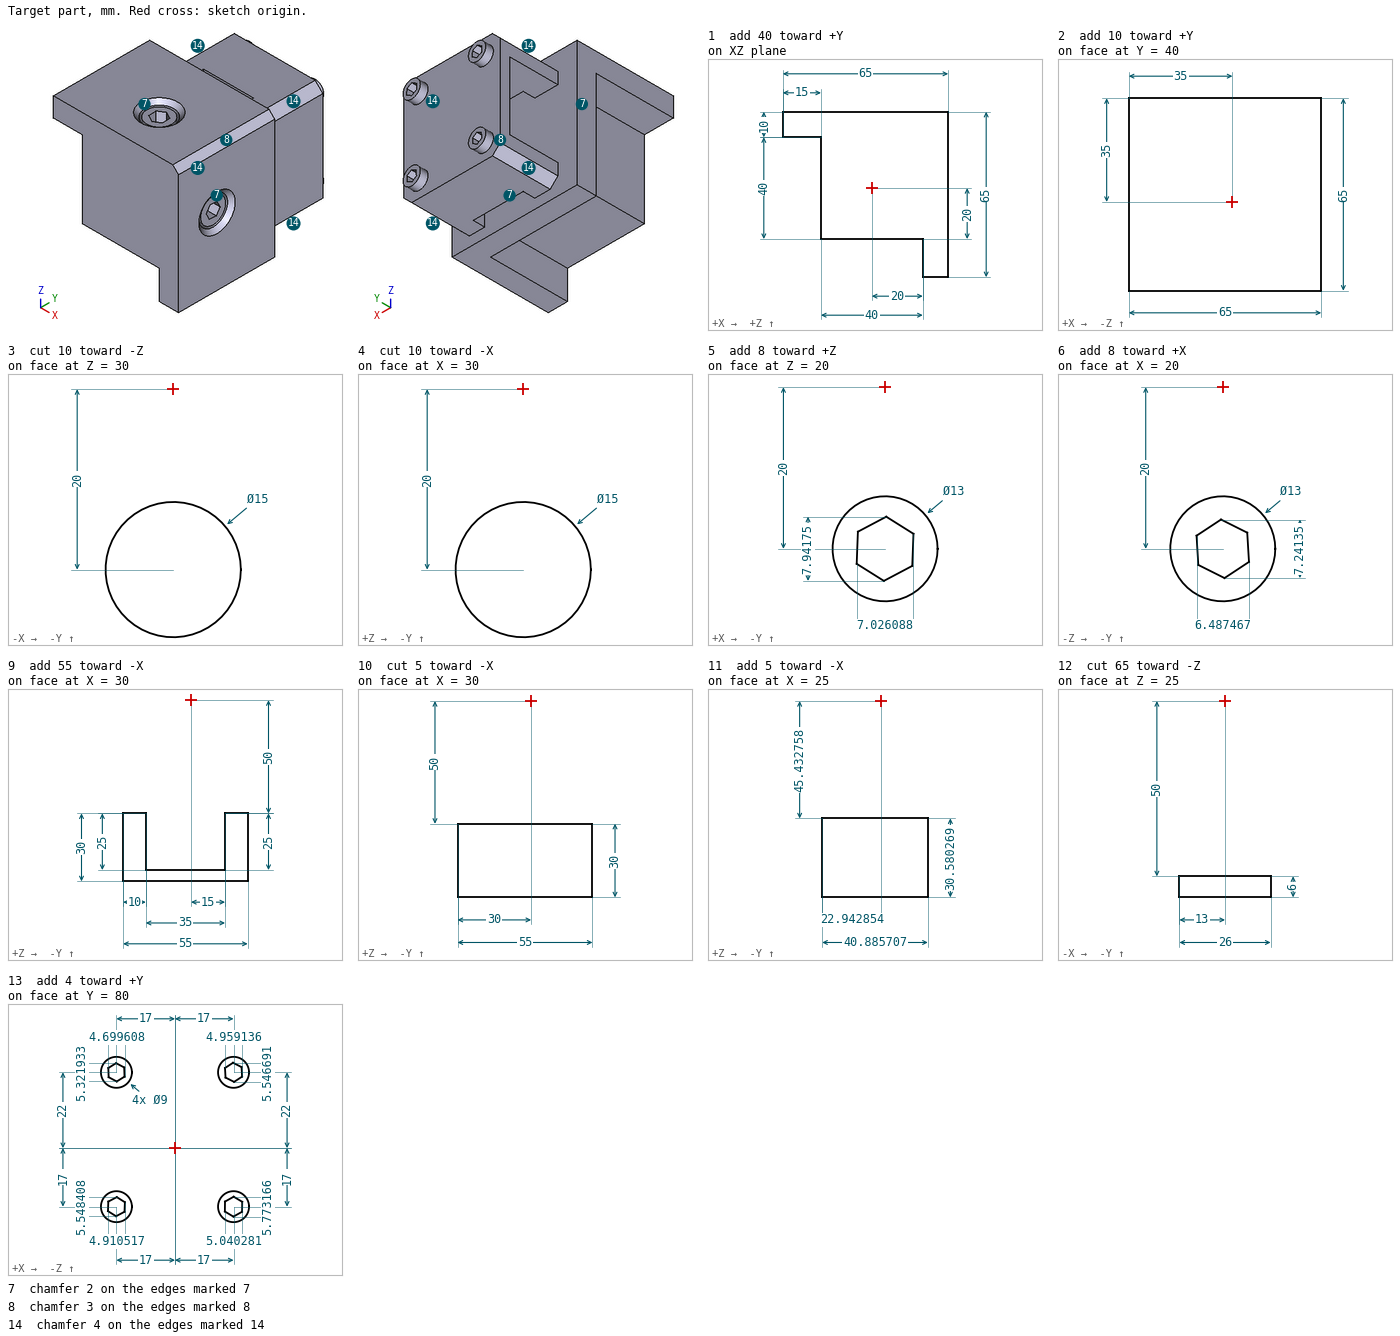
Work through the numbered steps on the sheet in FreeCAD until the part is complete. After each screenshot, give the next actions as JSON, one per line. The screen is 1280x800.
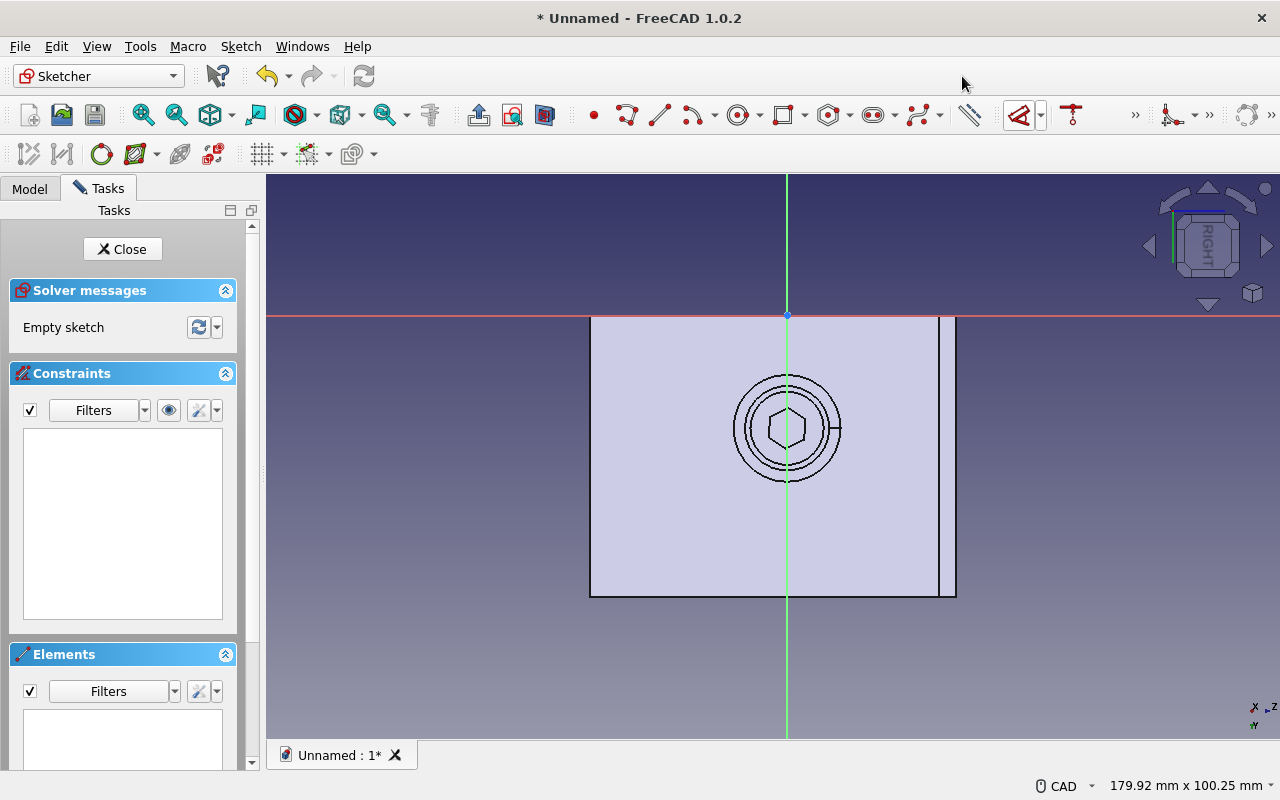
{"action": "scroll", "coordinate": [395, 202], "scroll_direction": "down", "scroll_amount": 1}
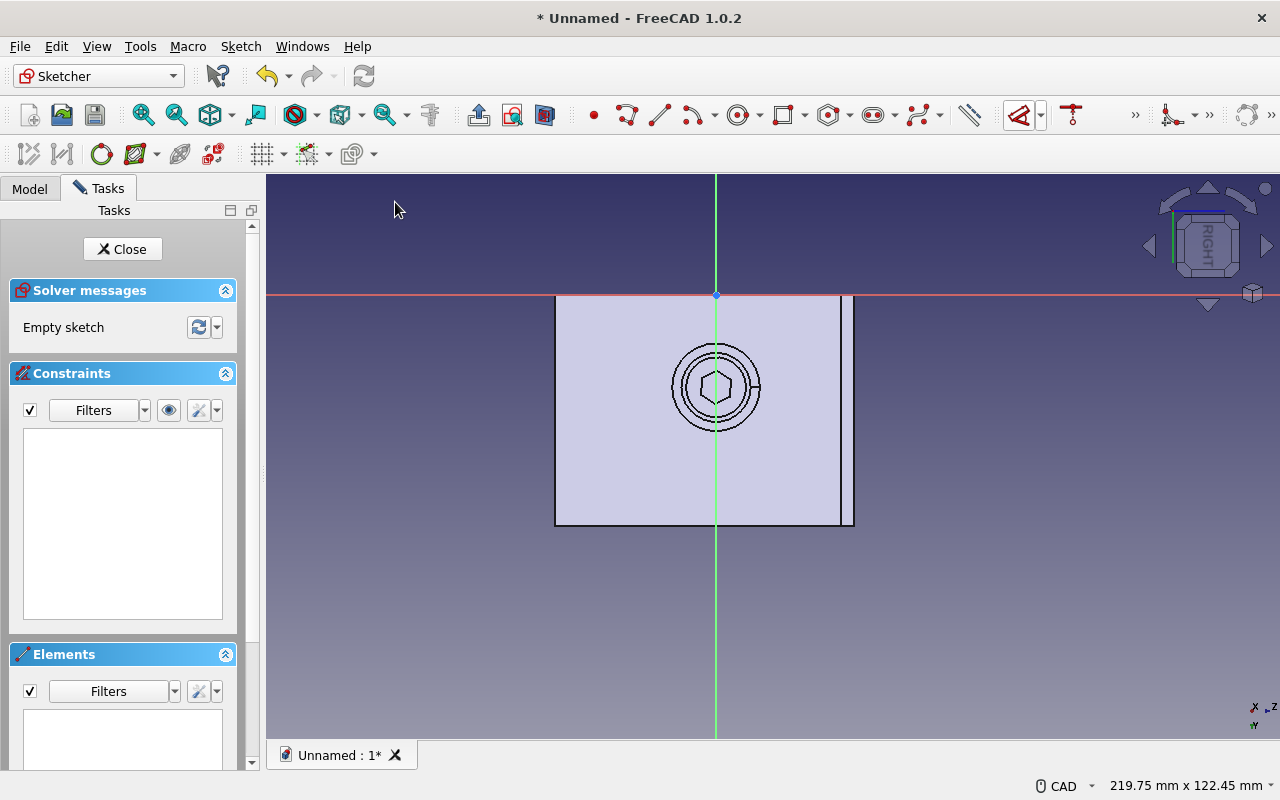
{"action": "left_click", "coordinate": [627, 116]}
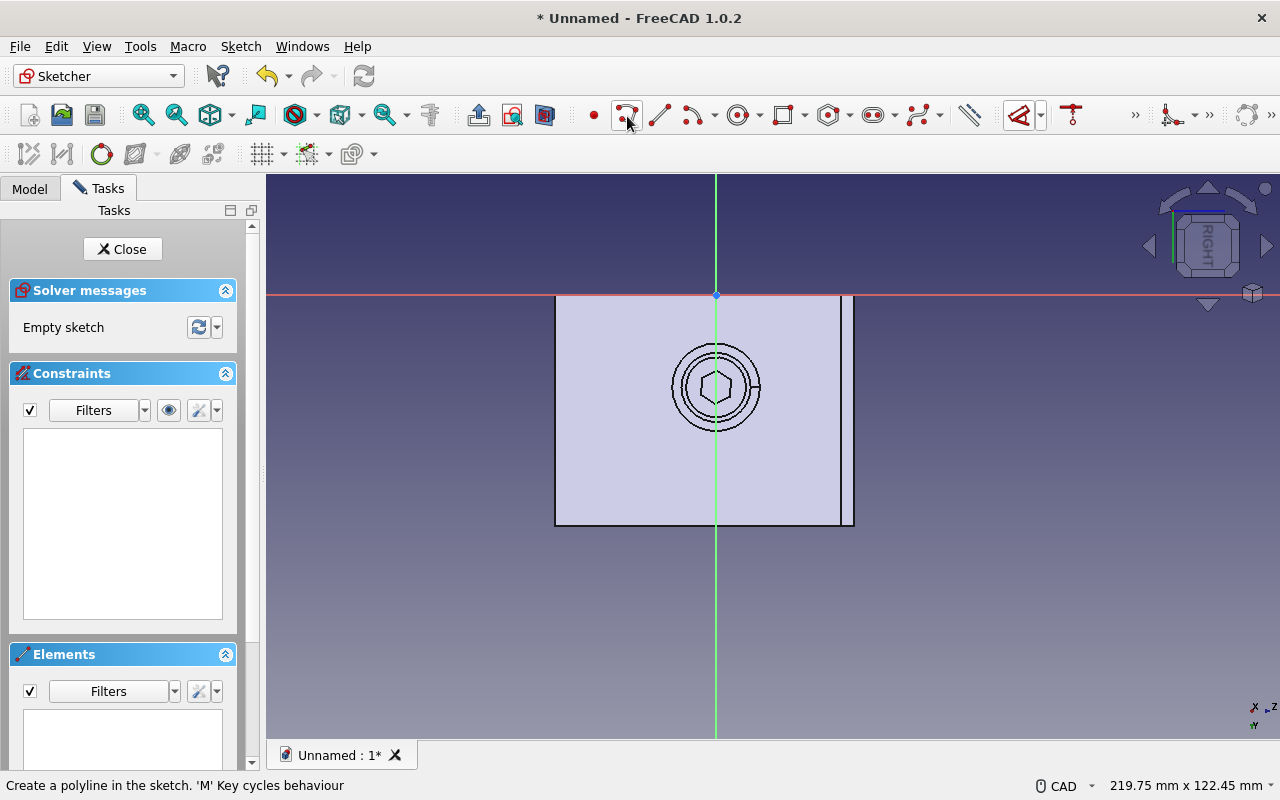
{"action": "left_click", "coordinate": [785, 526]}
{"action": "left_click", "coordinate": [785, 641]}
{"action": "left_click", "coordinate": [624, 641]}
{"action": "left_click", "coordinate": [624, 526]}
{"action": "left_click", "coordinate": [578, 526]}
{"action": "left_click", "coordinate": [578, 664]}
{"action": "left_click", "coordinate": [831, 664]}
{"action": "left_click", "coordinate": [831, 526]}
{"action": "left_click", "coordinate": [785, 527]}
{"action": "key", "text": "Escape"}
{"action": "key", "text": "Escape"}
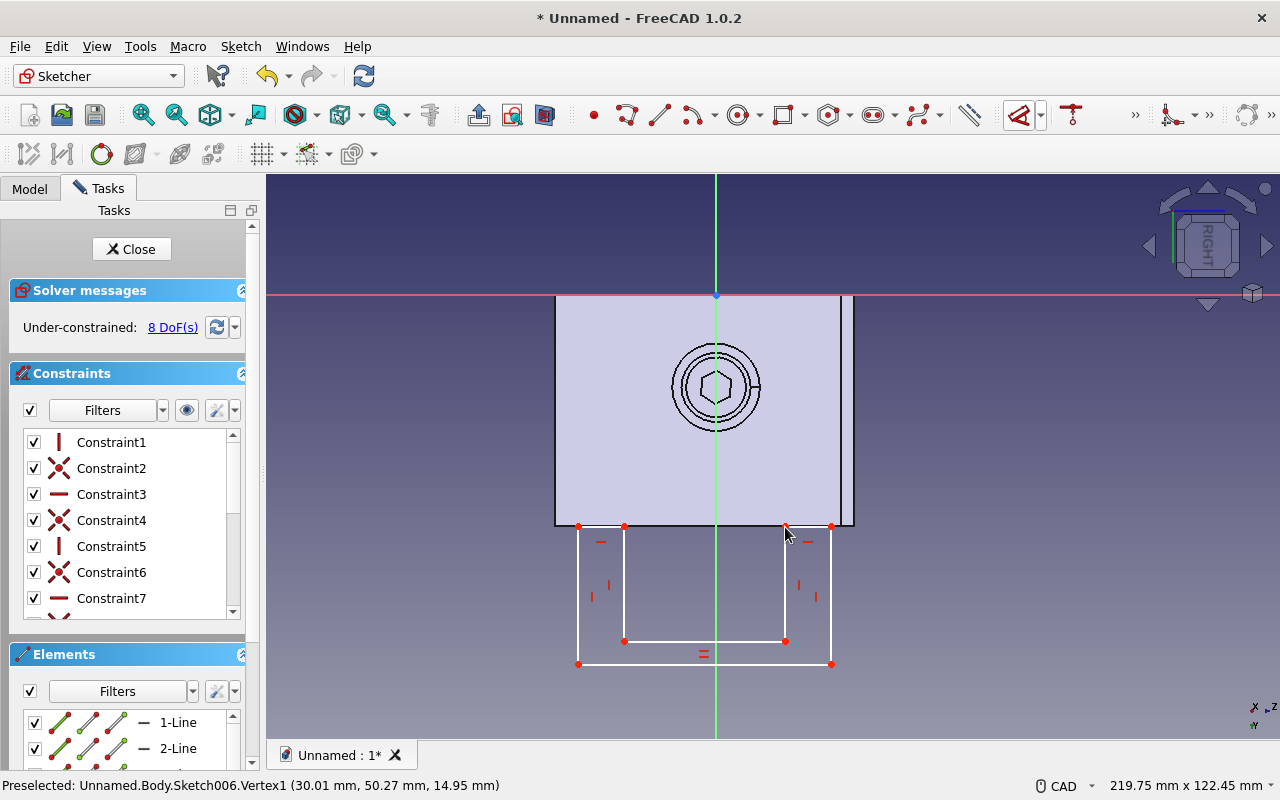
{"action": "left_click", "coordinate": [785, 561]}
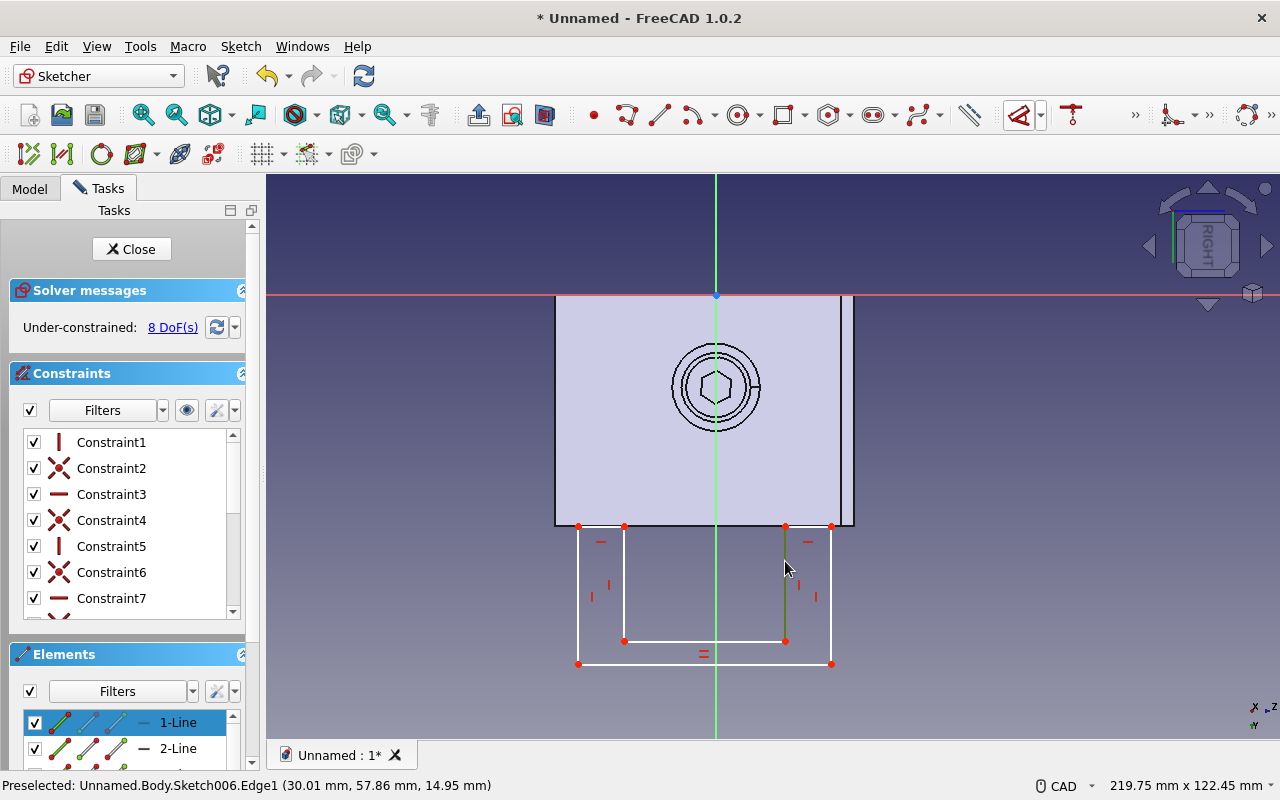
{"action": "left_click", "coordinate": [1040, 116]}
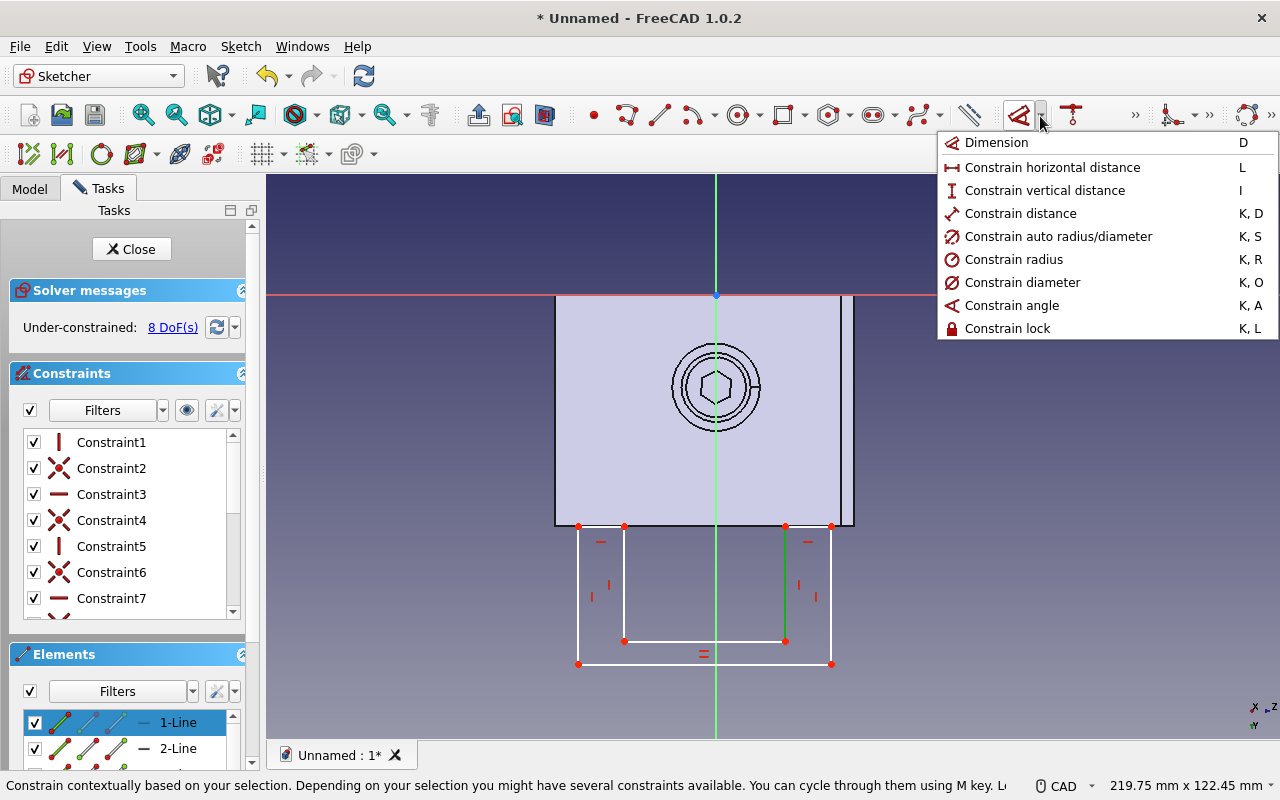
{"action": "left_click", "coordinate": [1108, 190]}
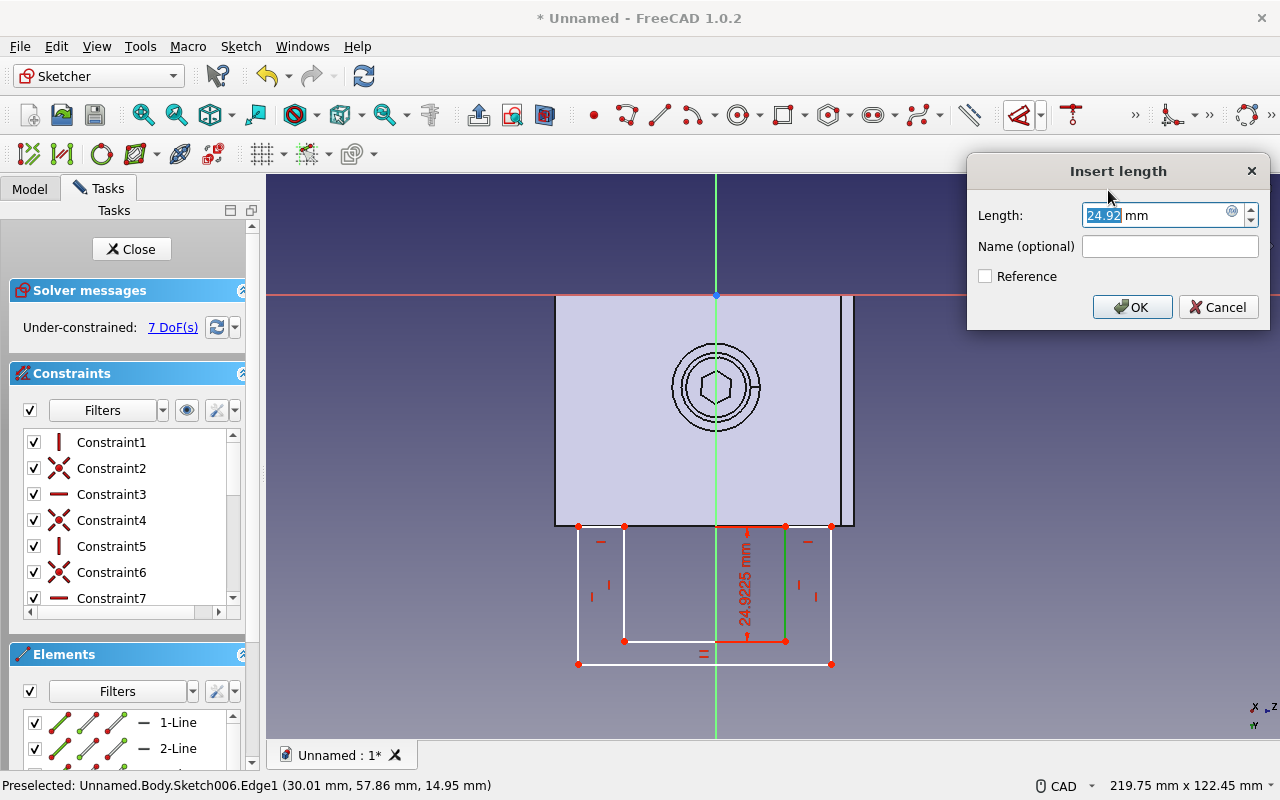
{"action": "type", "text": "25"}
{"action": "key", "text": "Return"}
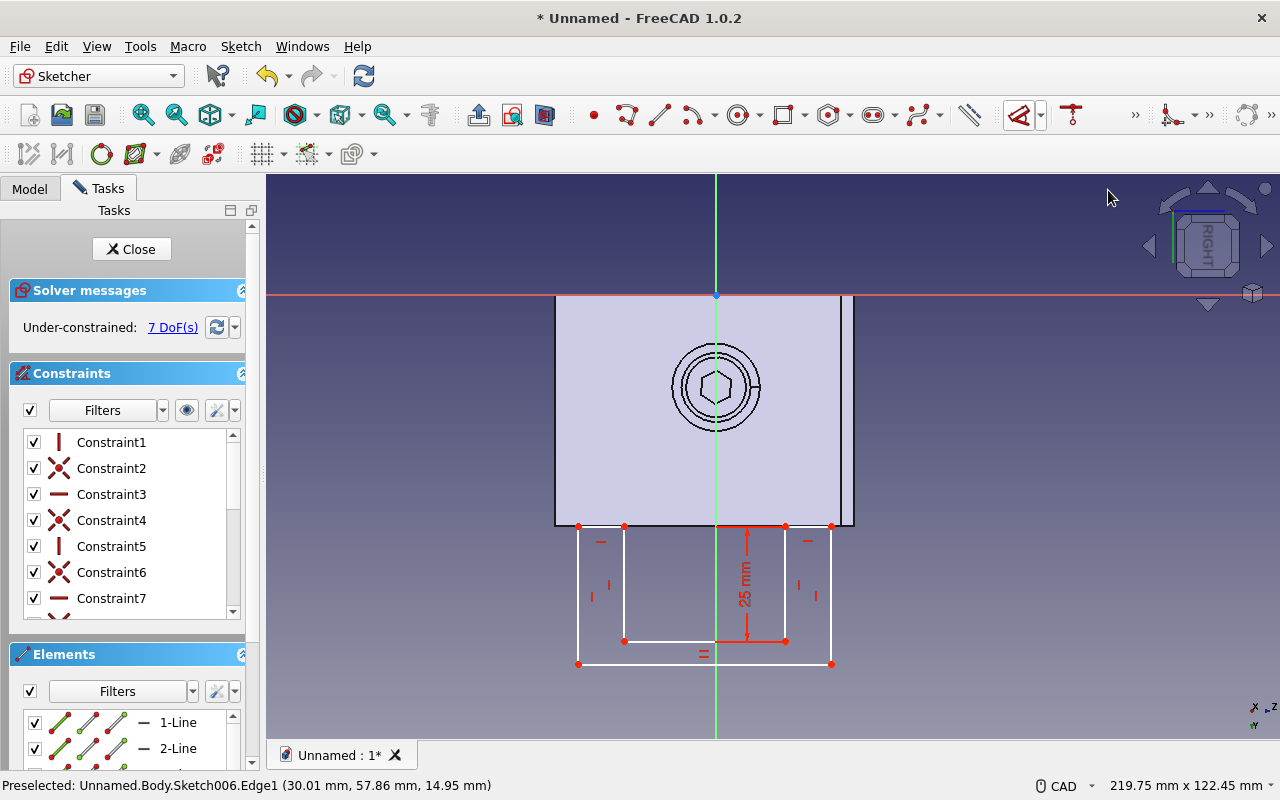
{"action": "left_click", "coordinate": [737, 642]}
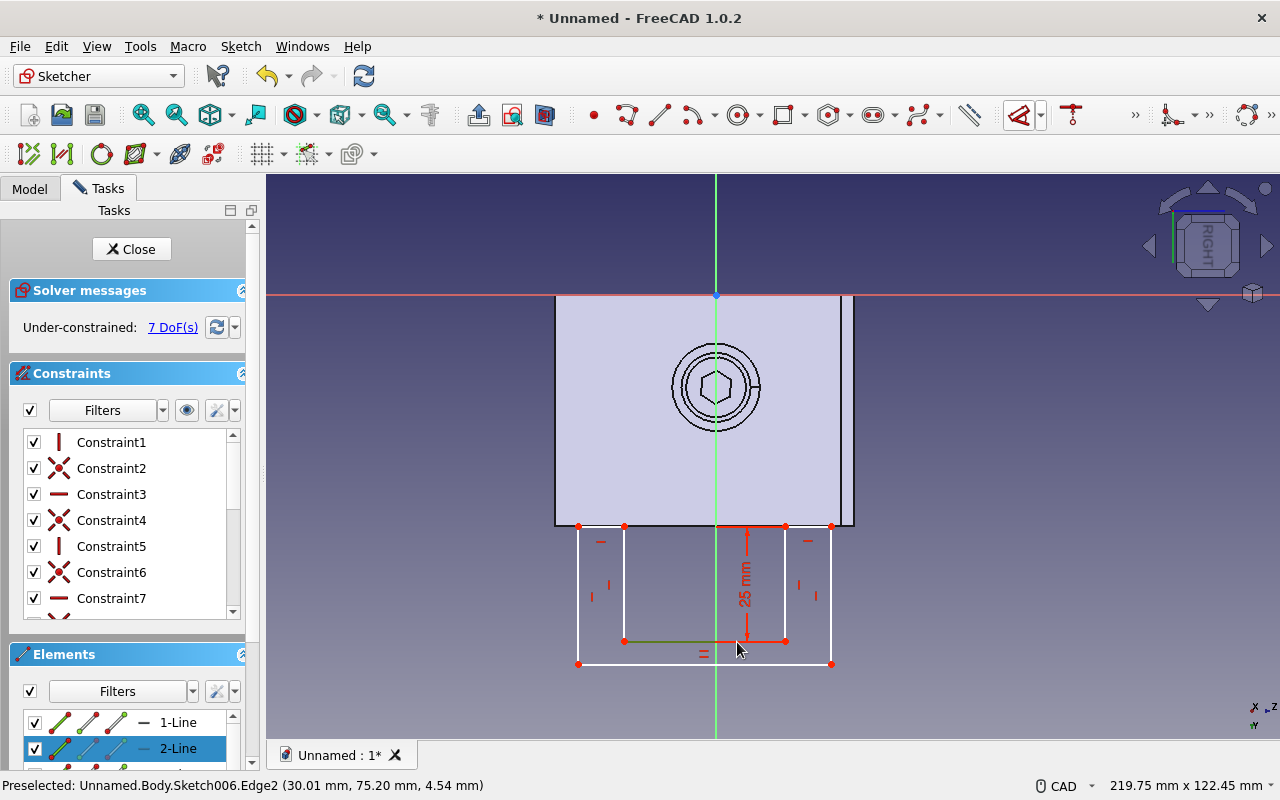
{"action": "left_click", "coordinate": [1040, 116]}